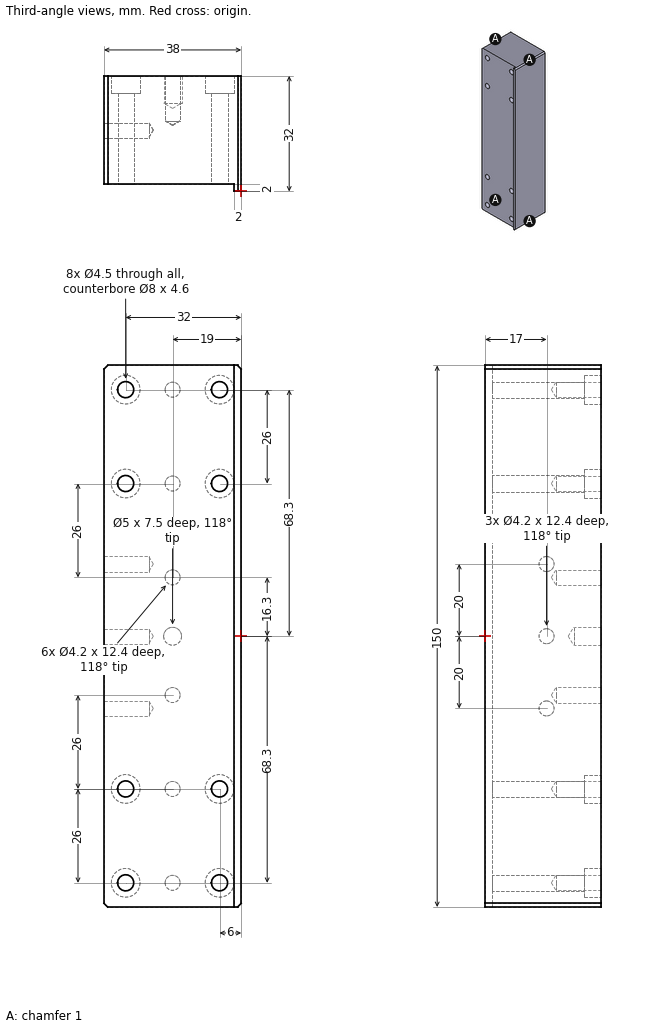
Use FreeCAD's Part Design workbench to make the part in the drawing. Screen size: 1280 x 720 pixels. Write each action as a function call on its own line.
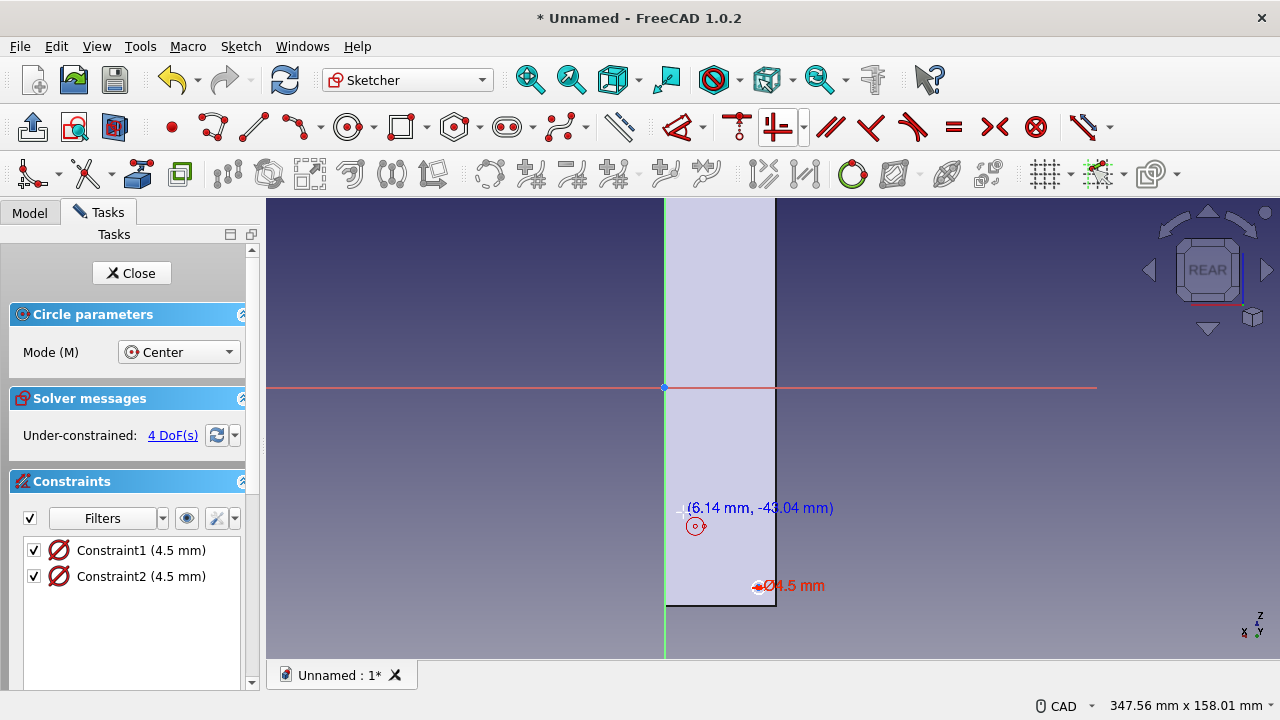
click(682, 511)
move(687, 506)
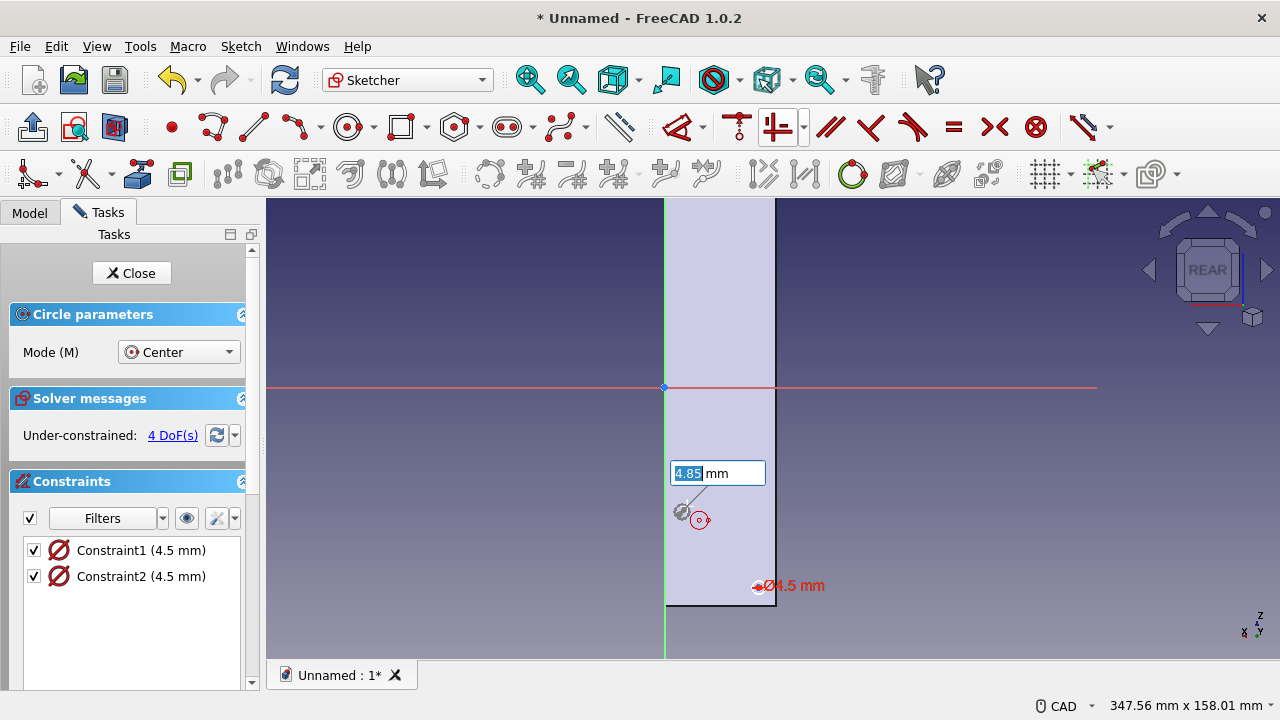
text(4.5)
key(Return)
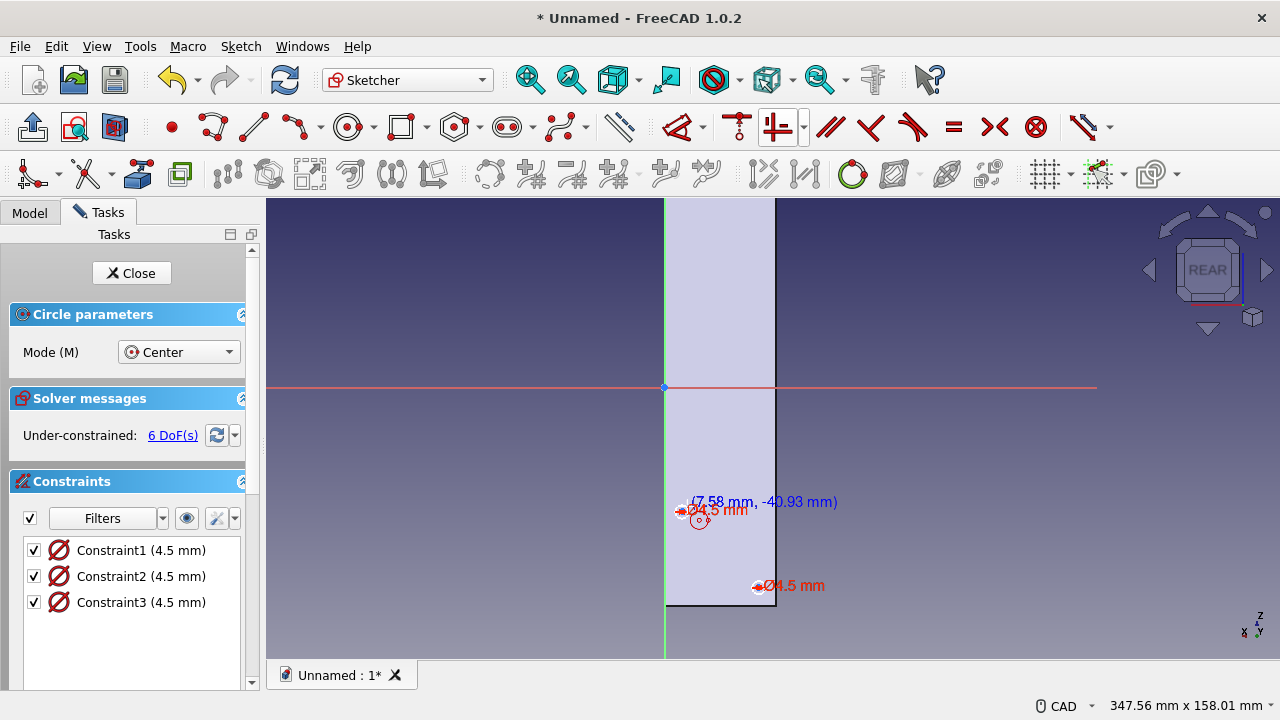
scroll(758, 511, up, 7)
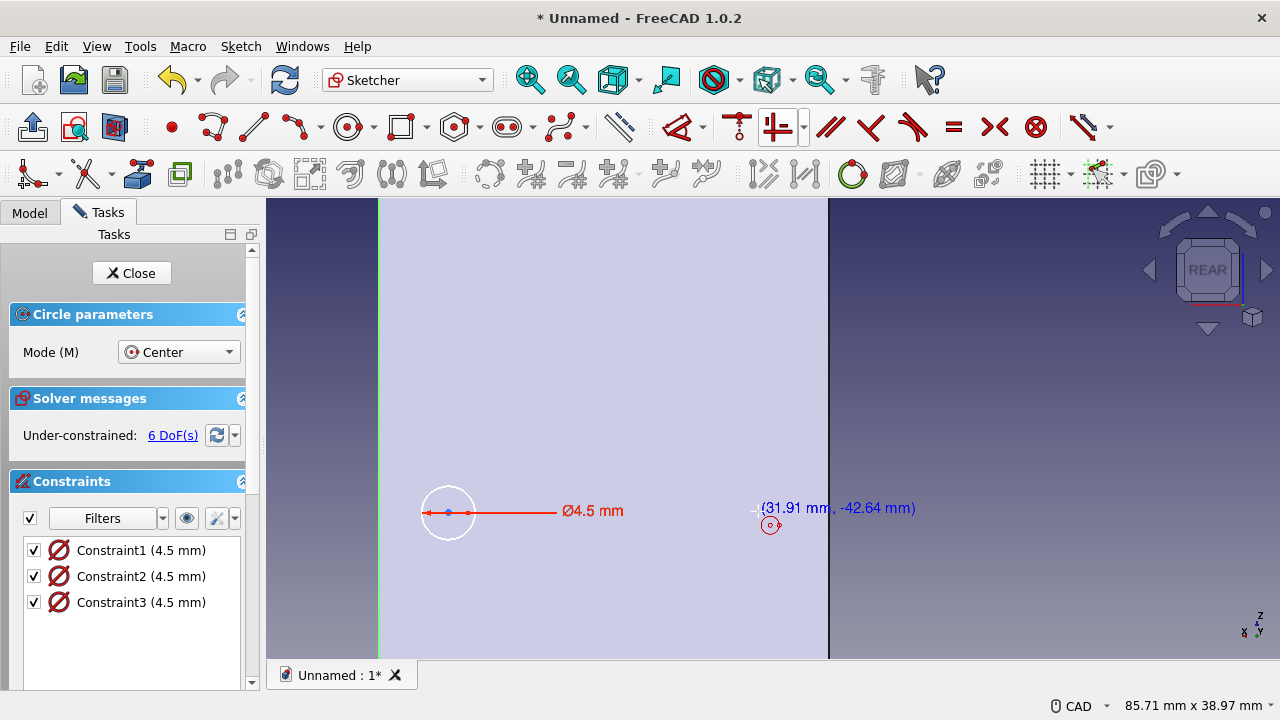
scroll(729, 512, down, 9)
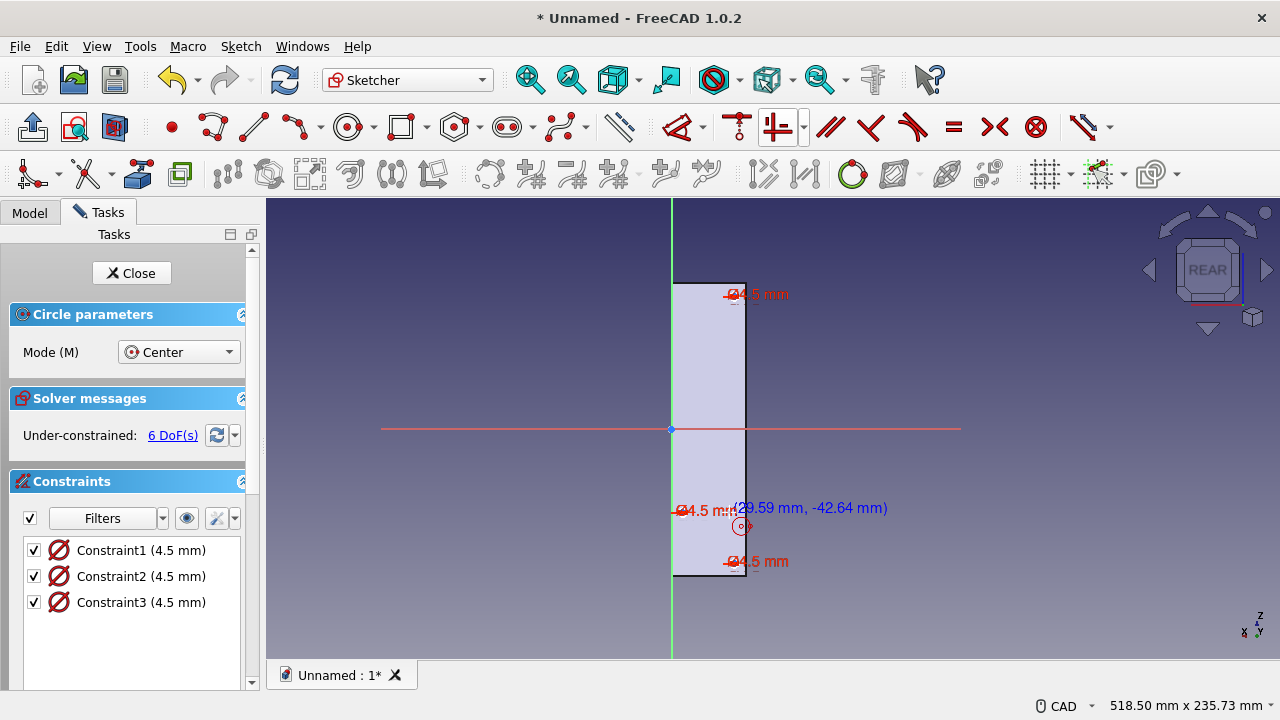
click(734, 512)
move(737, 509)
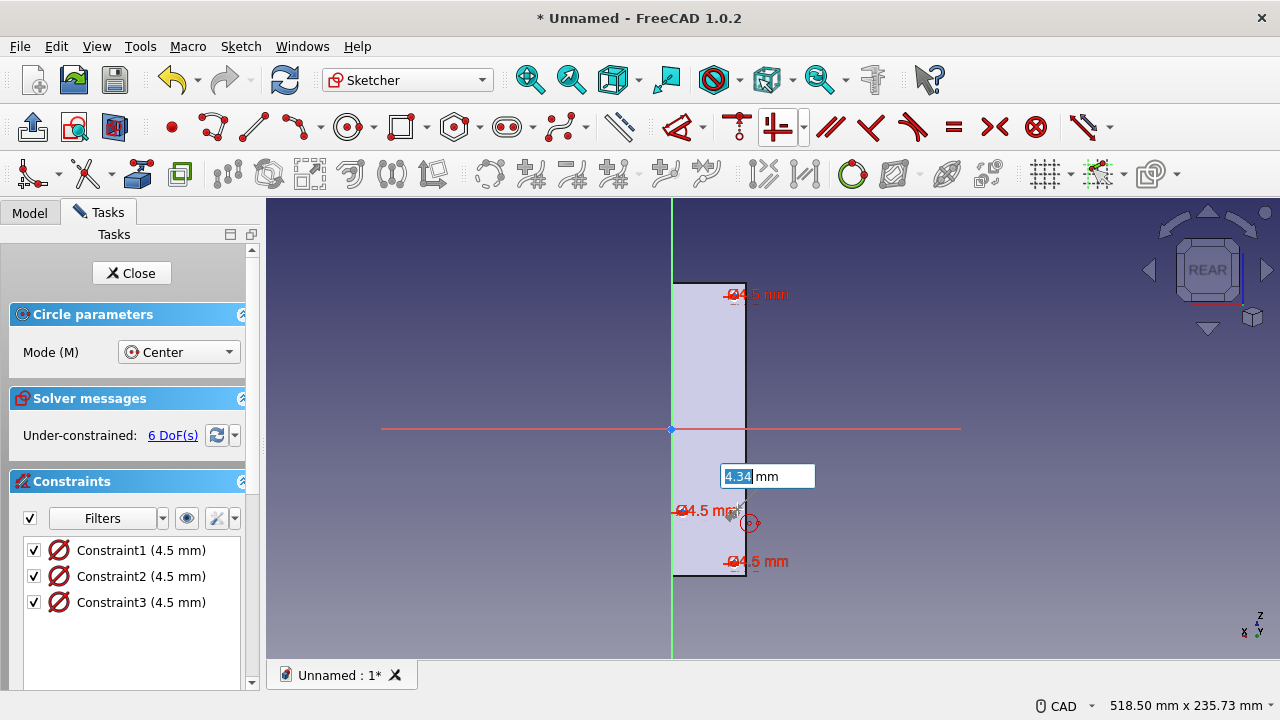
text(4.5)
key(Return)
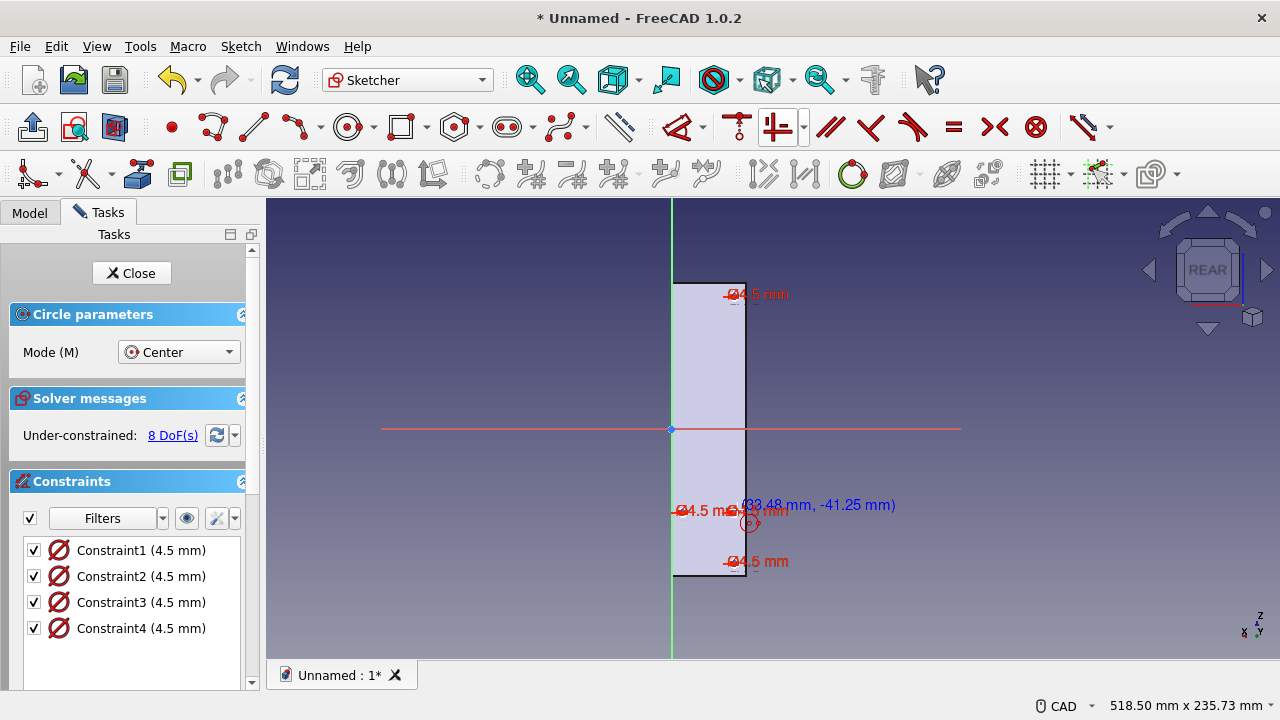
scroll(683, 563, up, 9)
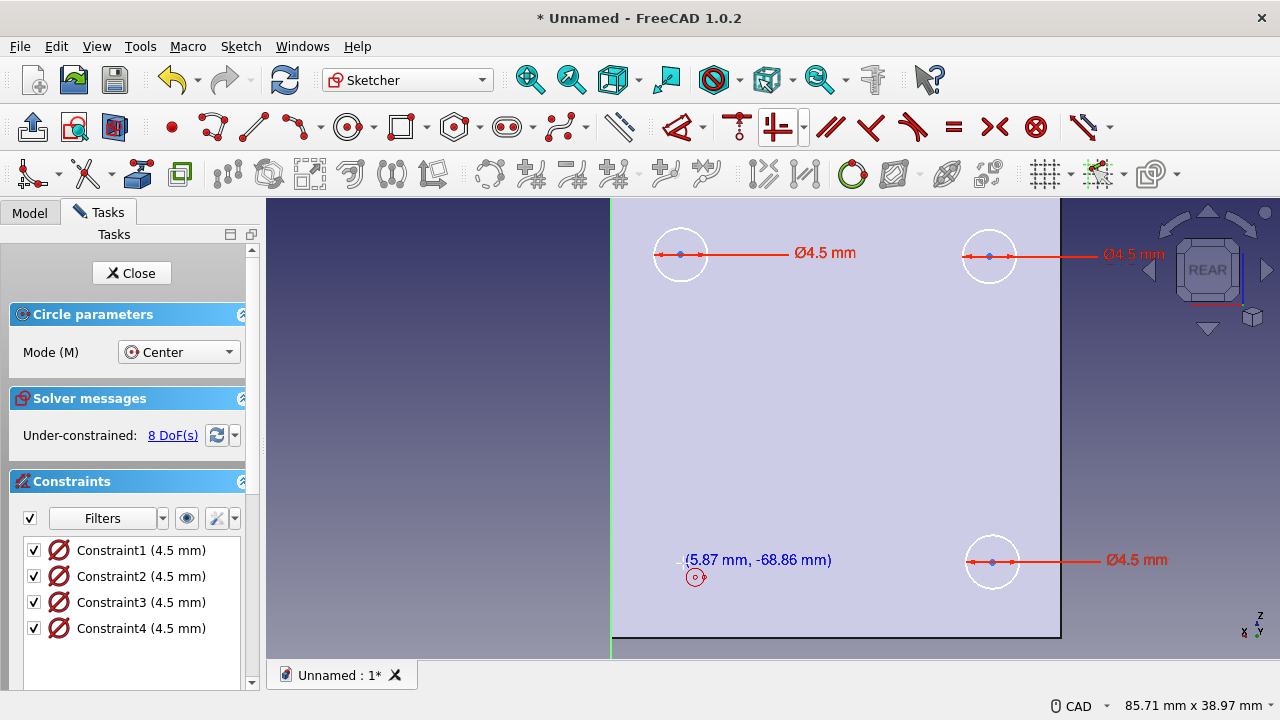
scroll(683, 563, down, 9)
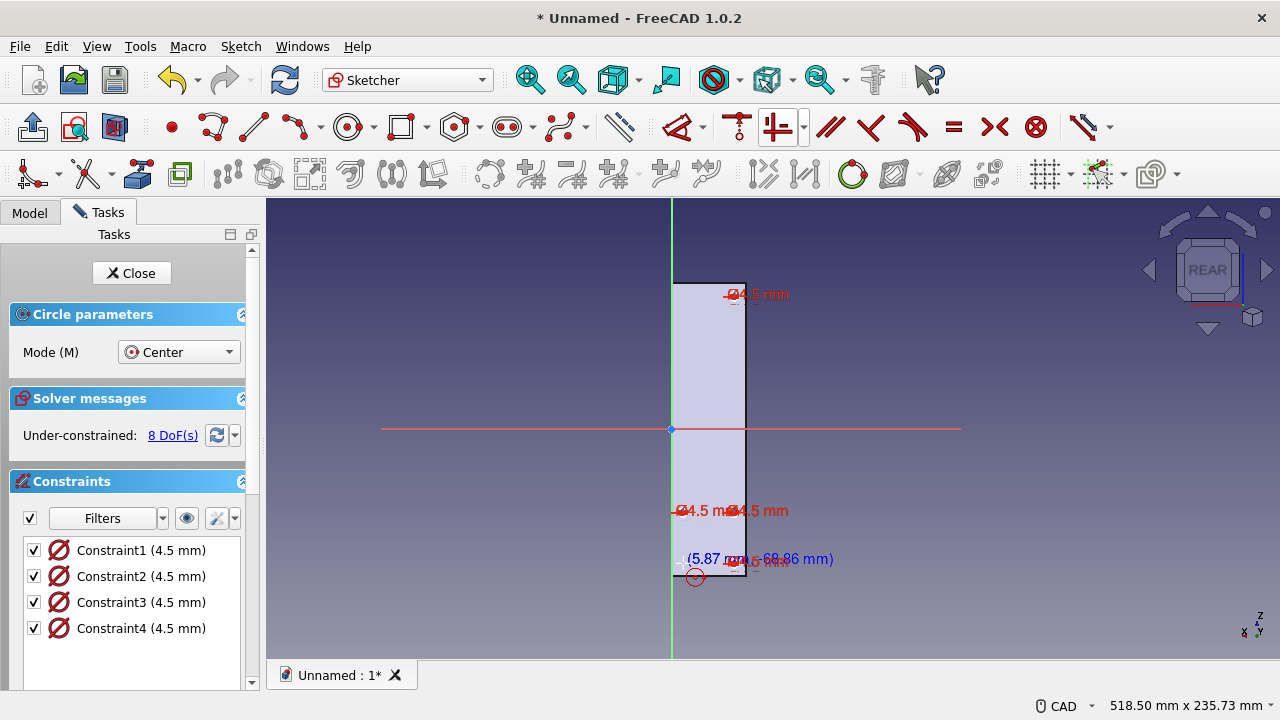
scroll(683, 563, up, 2)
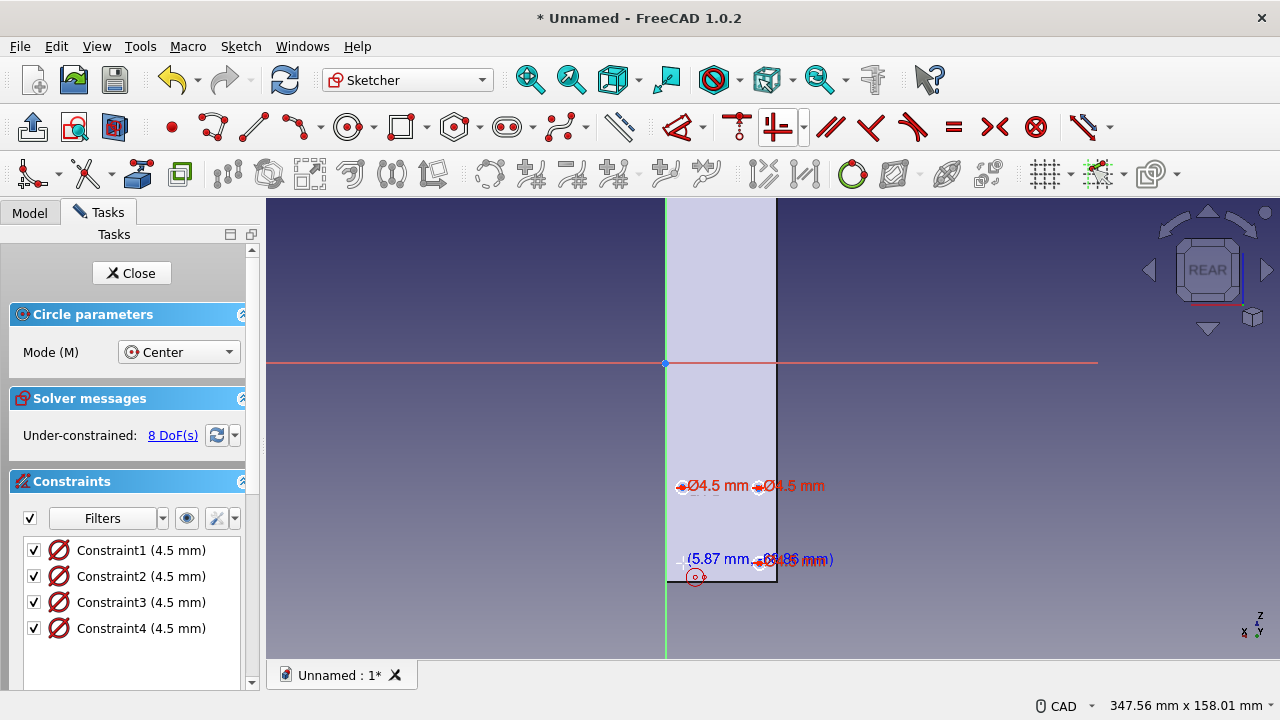
click(683, 562)
move(688, 558)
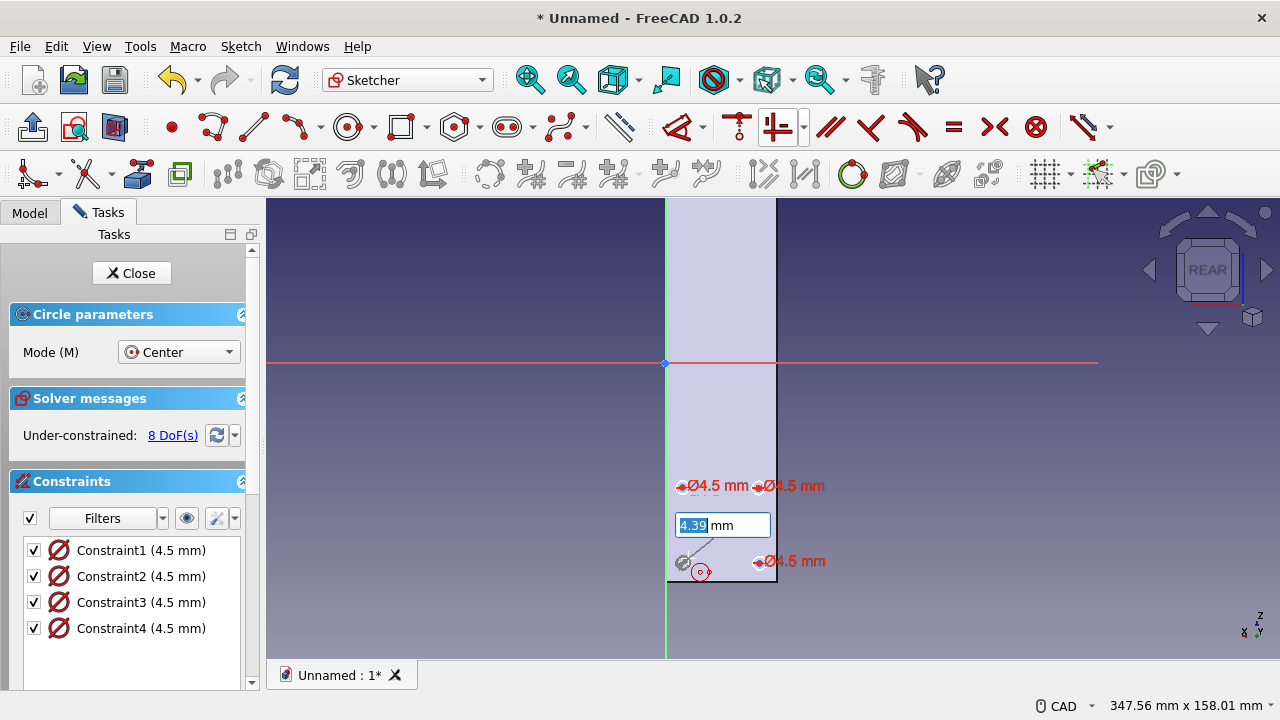
text(4.5)
key(Return)